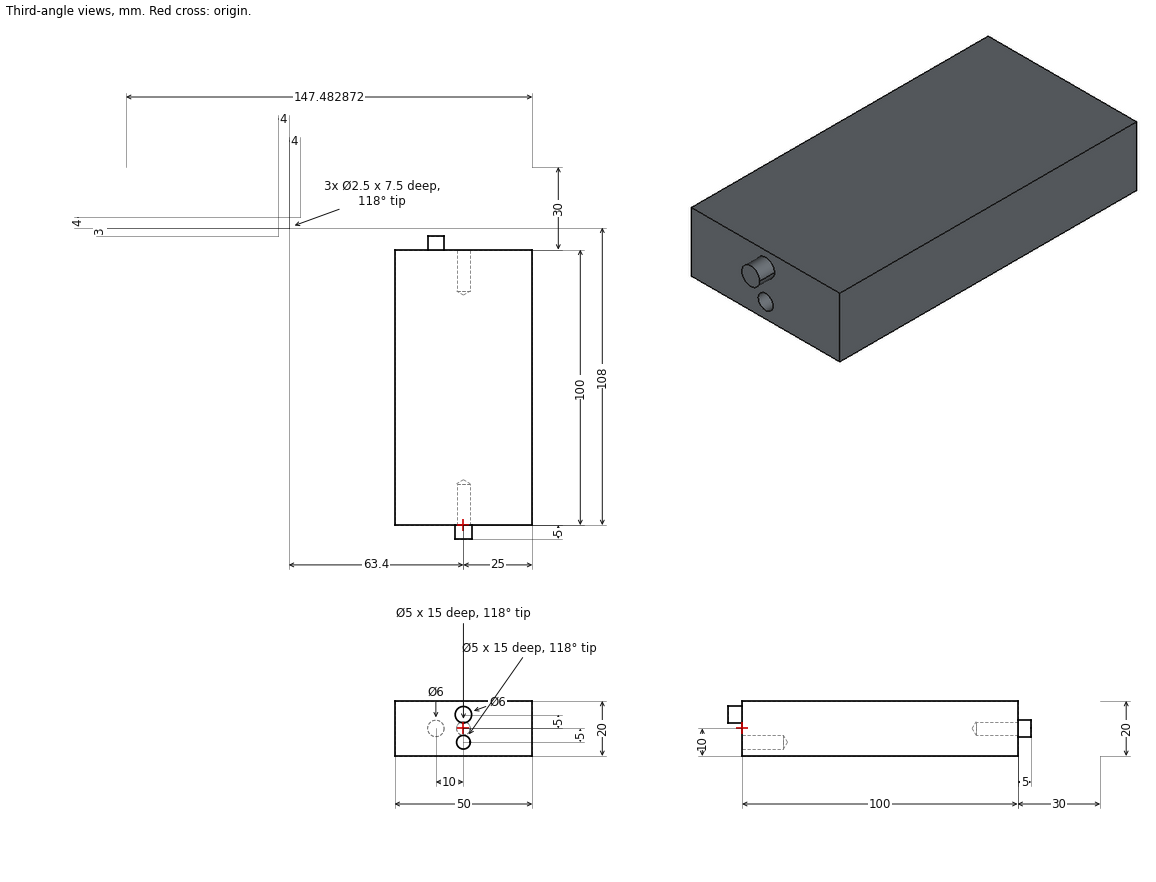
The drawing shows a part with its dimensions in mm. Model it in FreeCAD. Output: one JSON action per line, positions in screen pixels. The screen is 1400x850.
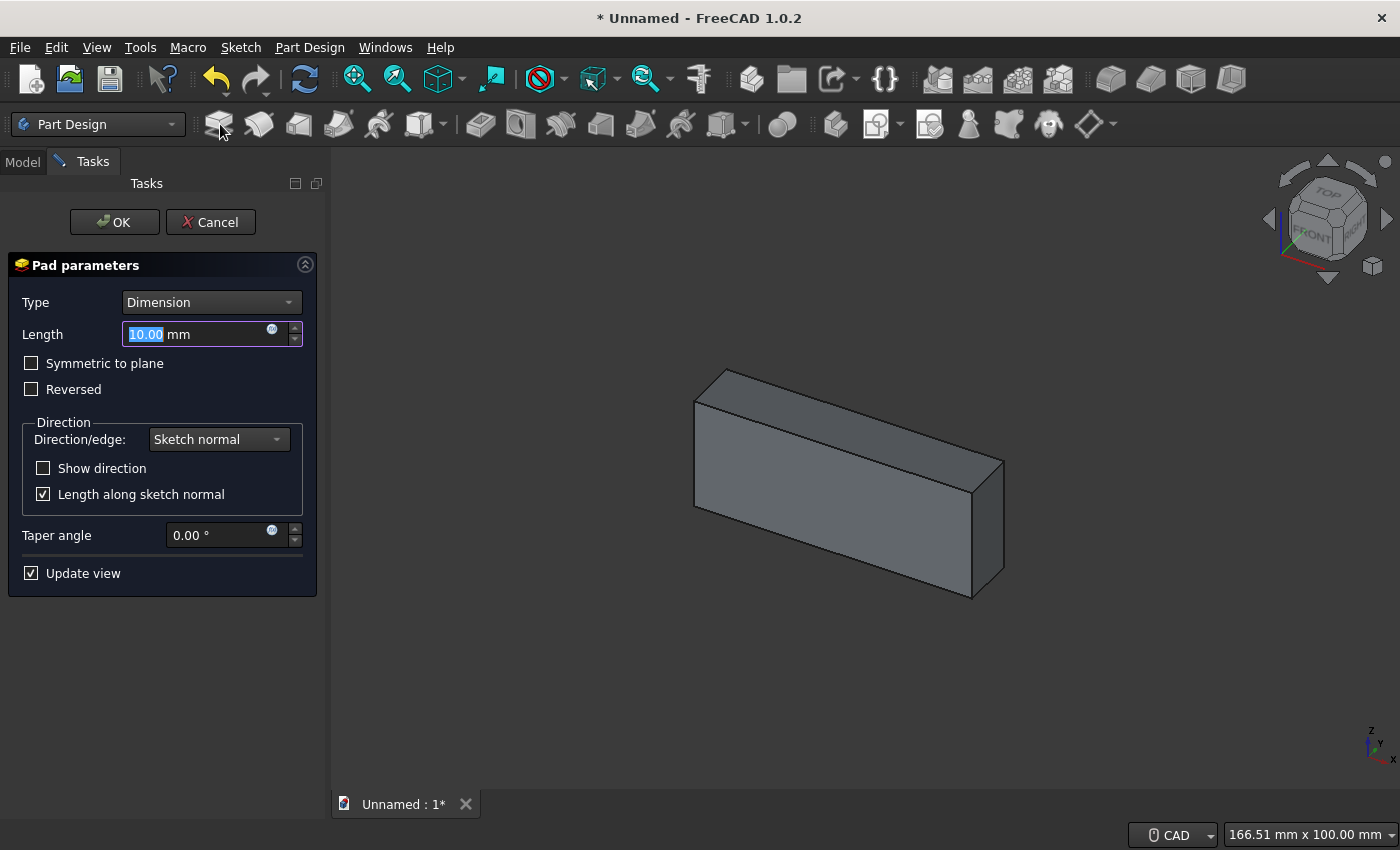
{"action": "type", "text": "100"}
{"action": "key", "text": "Tab"}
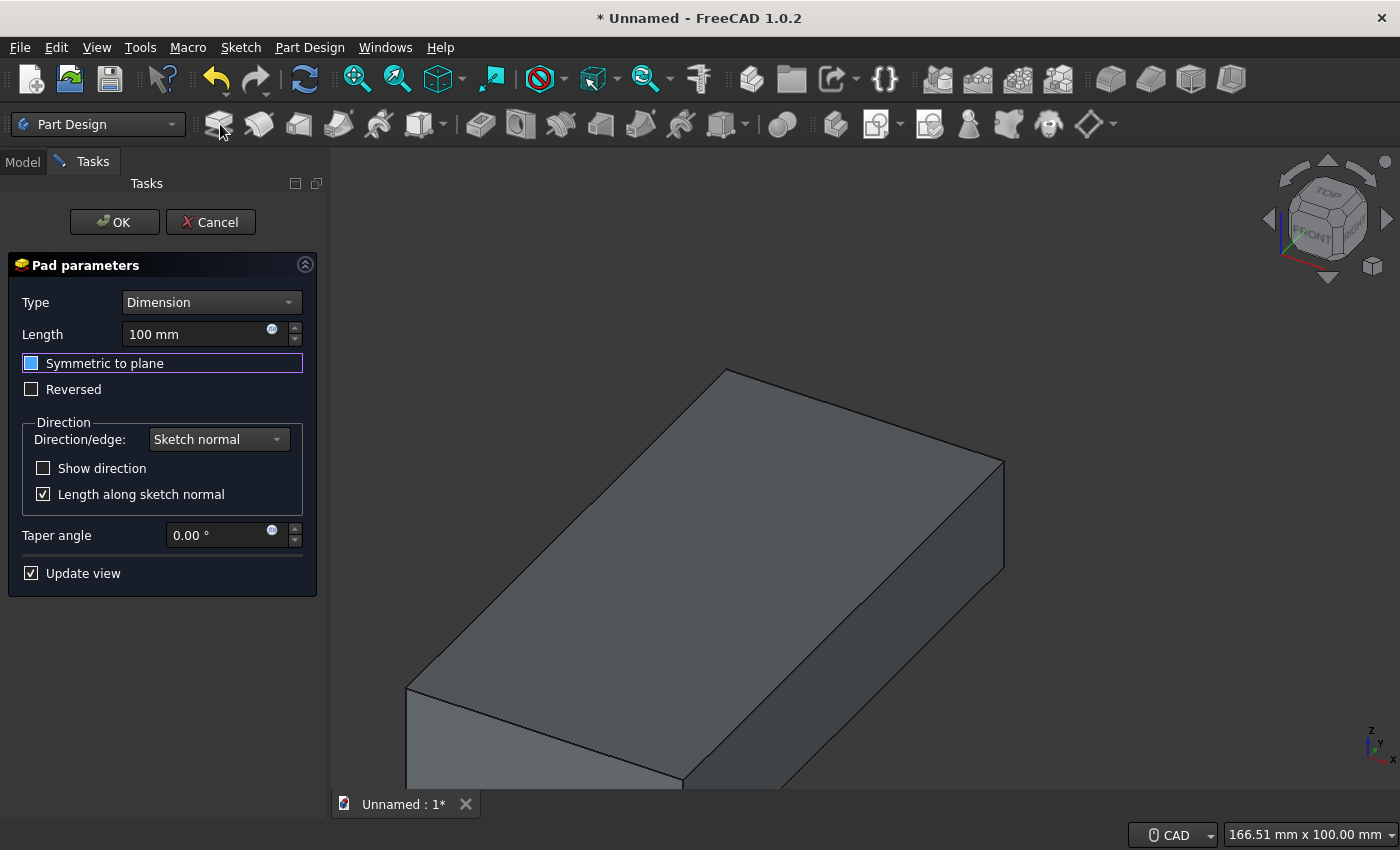
{"action": "left_click", "coordinate": [30, 389]}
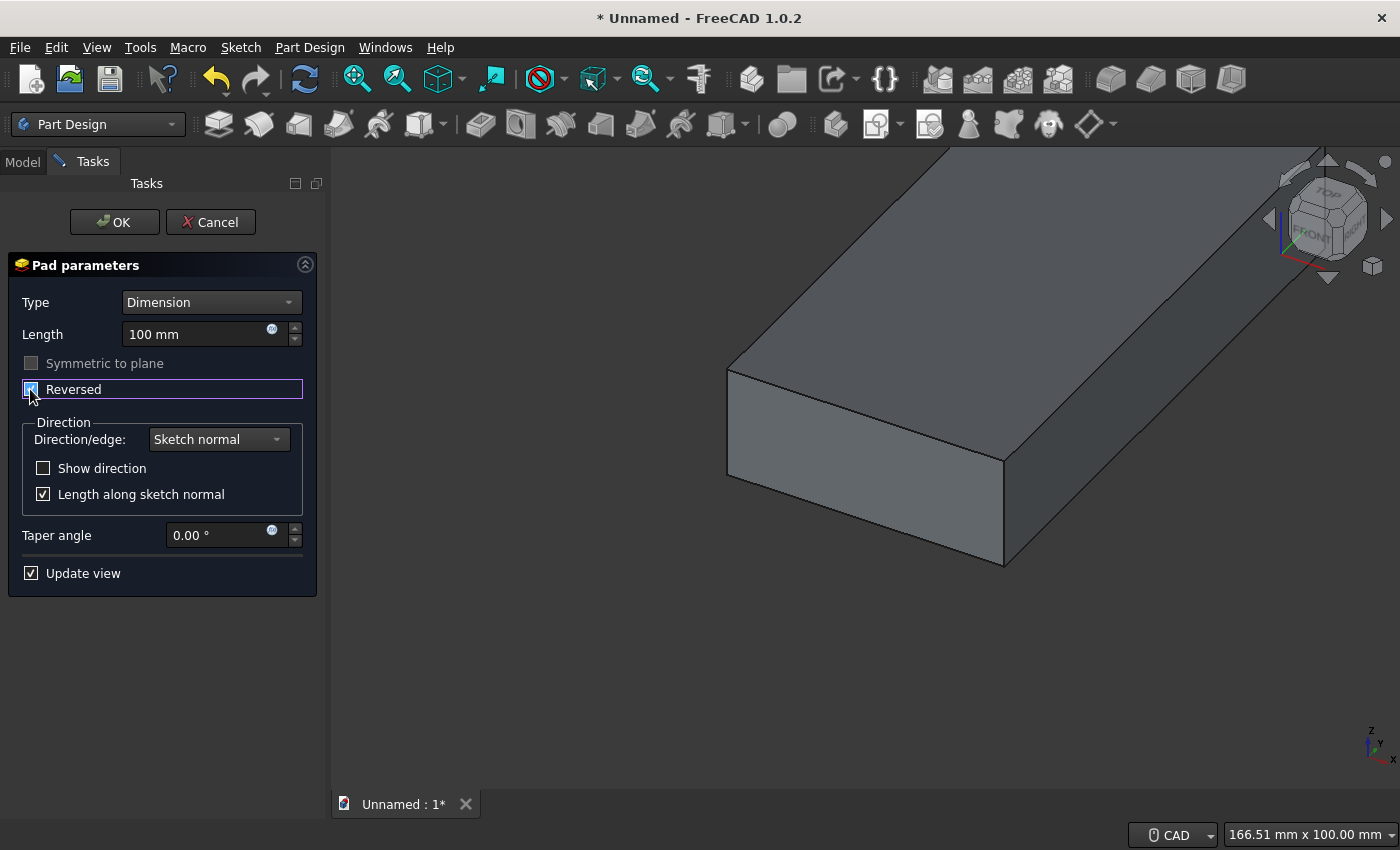
{"action": "left_click", "coordinate": [115, 222]}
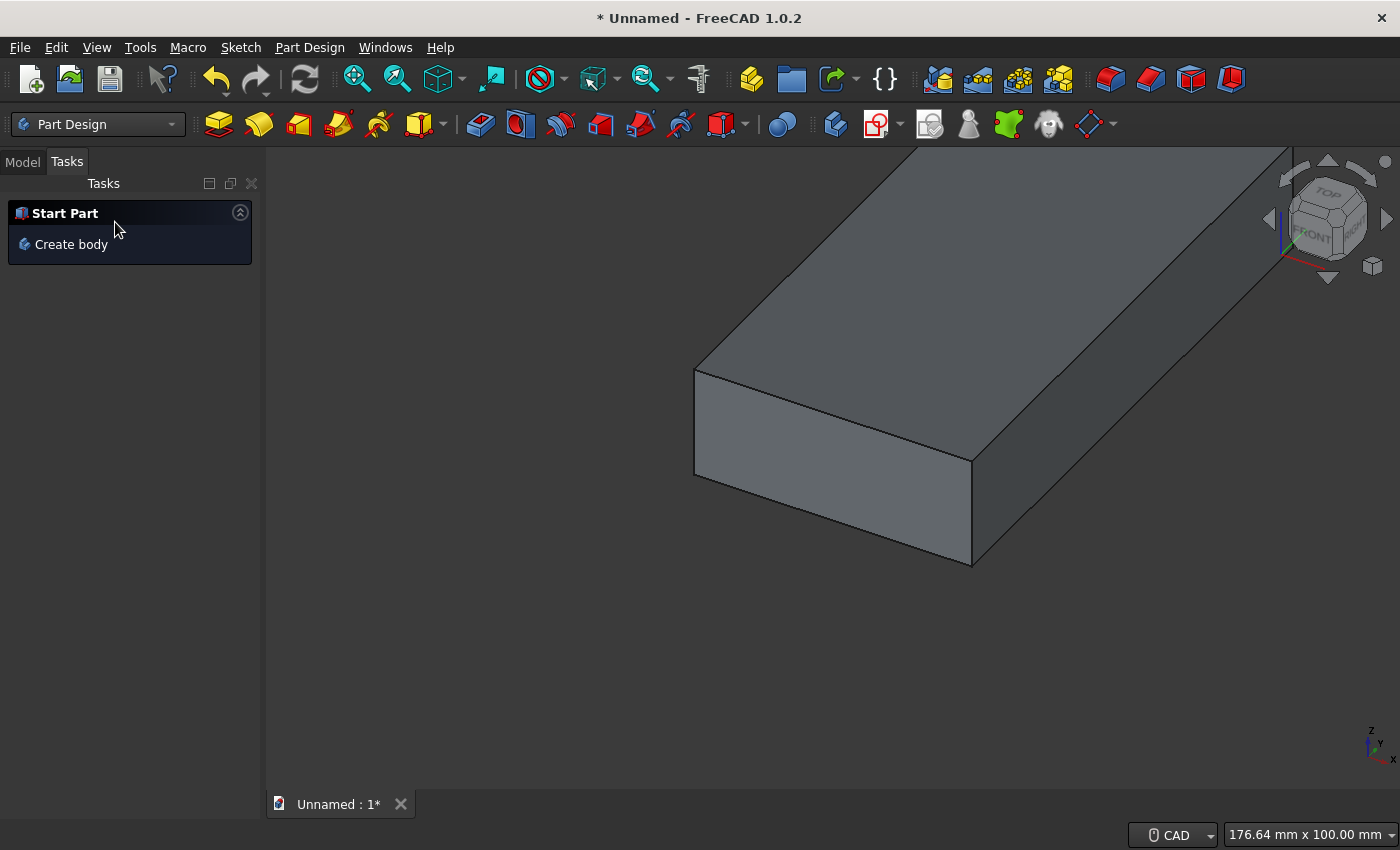
{"action": "key", "text": "v f"}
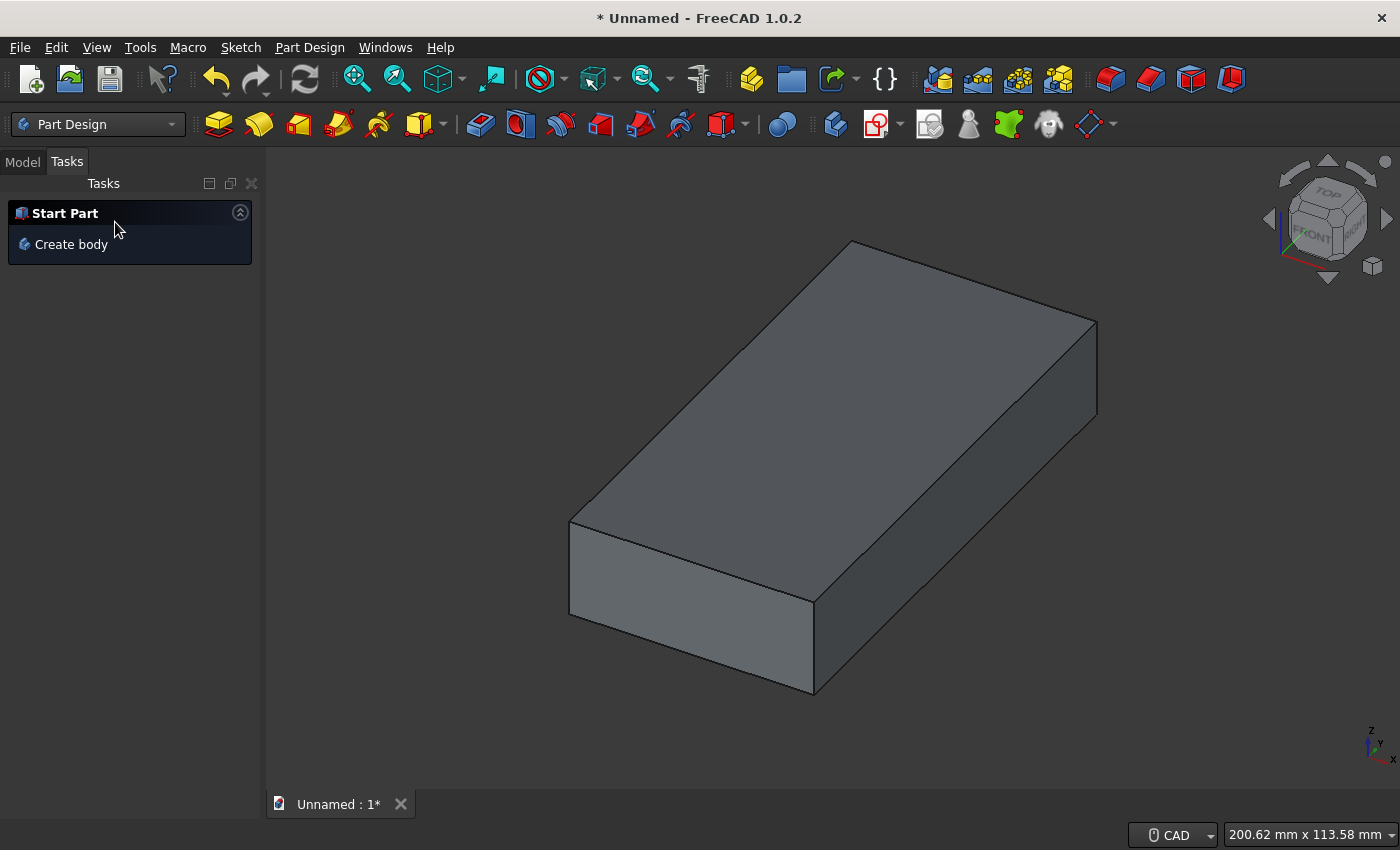
{"action": "left_click", "coordinate": [876, 124]}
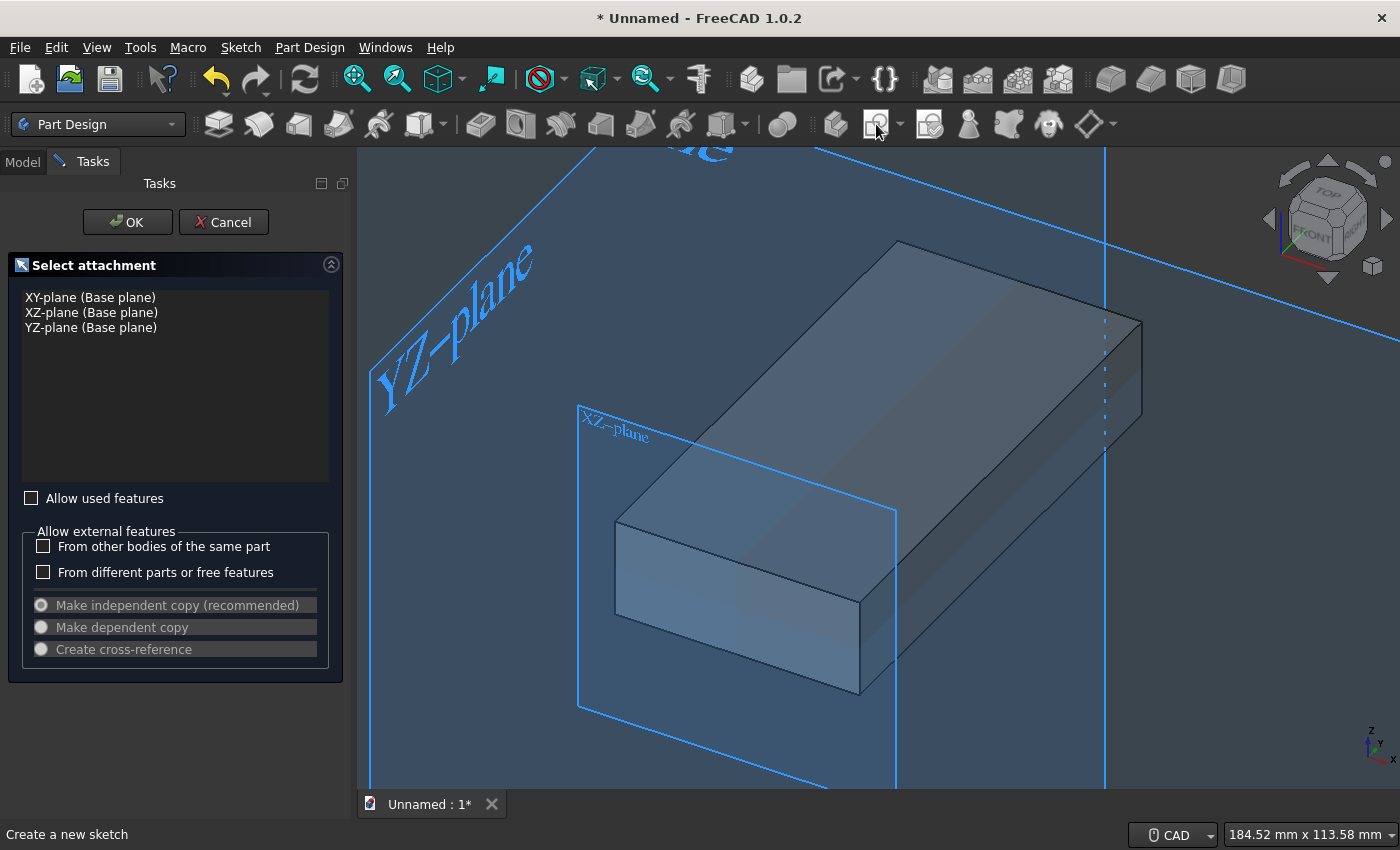
{"action": "left_click", "coordinate": [82, 312]}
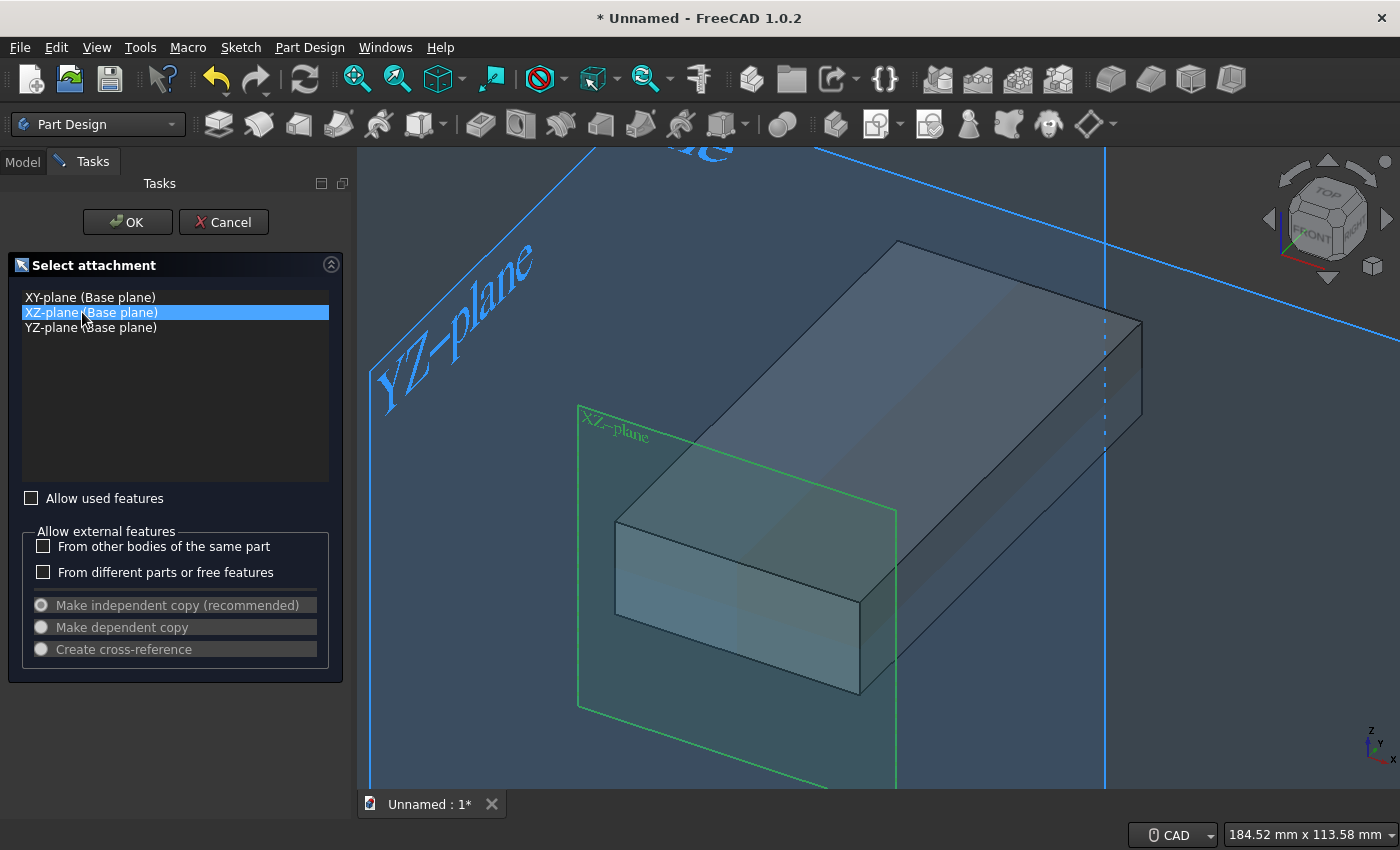
{"action": "left_click", "coordinate": [128, 222]}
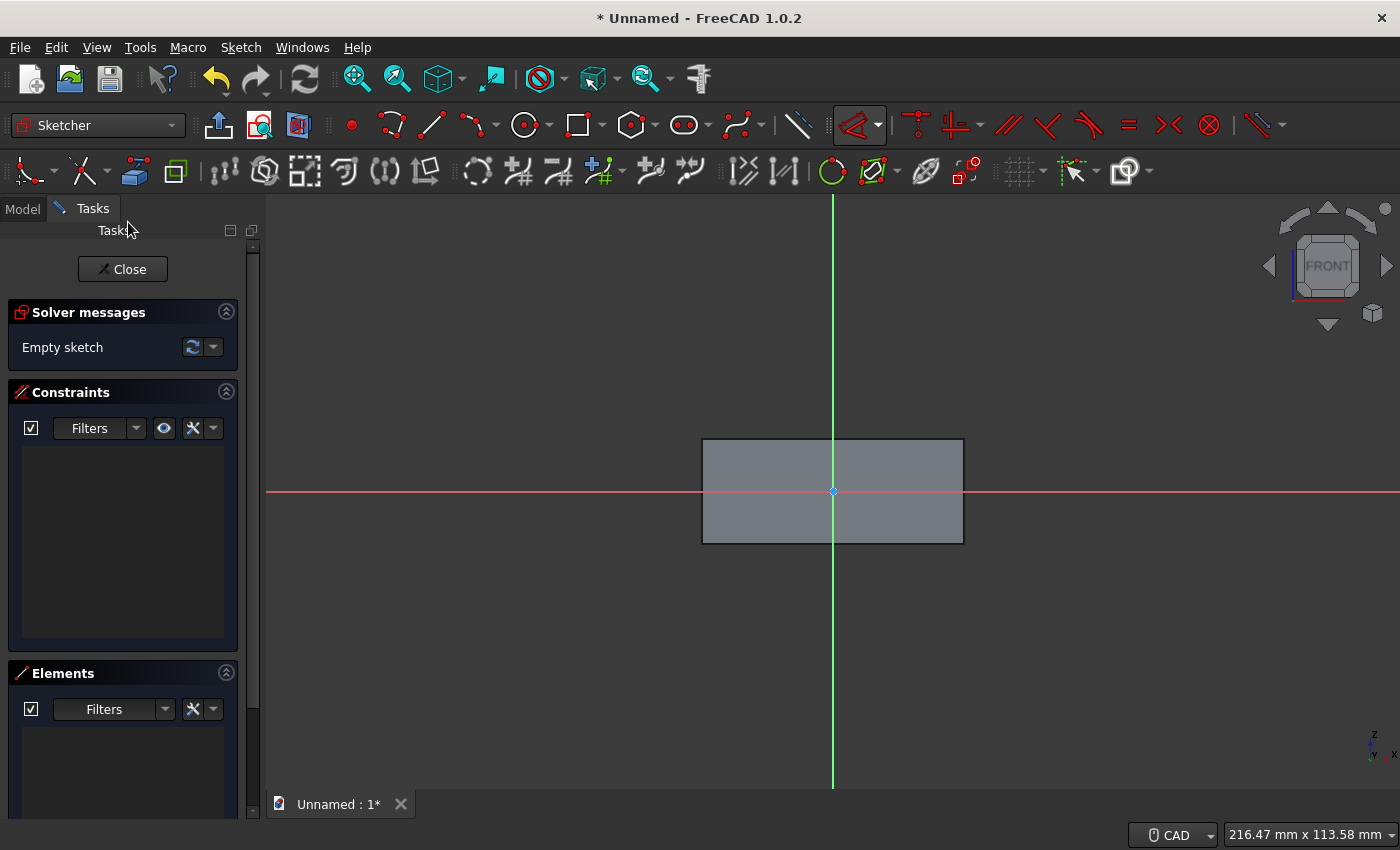
{"action": "scroll", "coordinate": [842, 468], "scroll_direction": "up", "scroll_amount": 11}